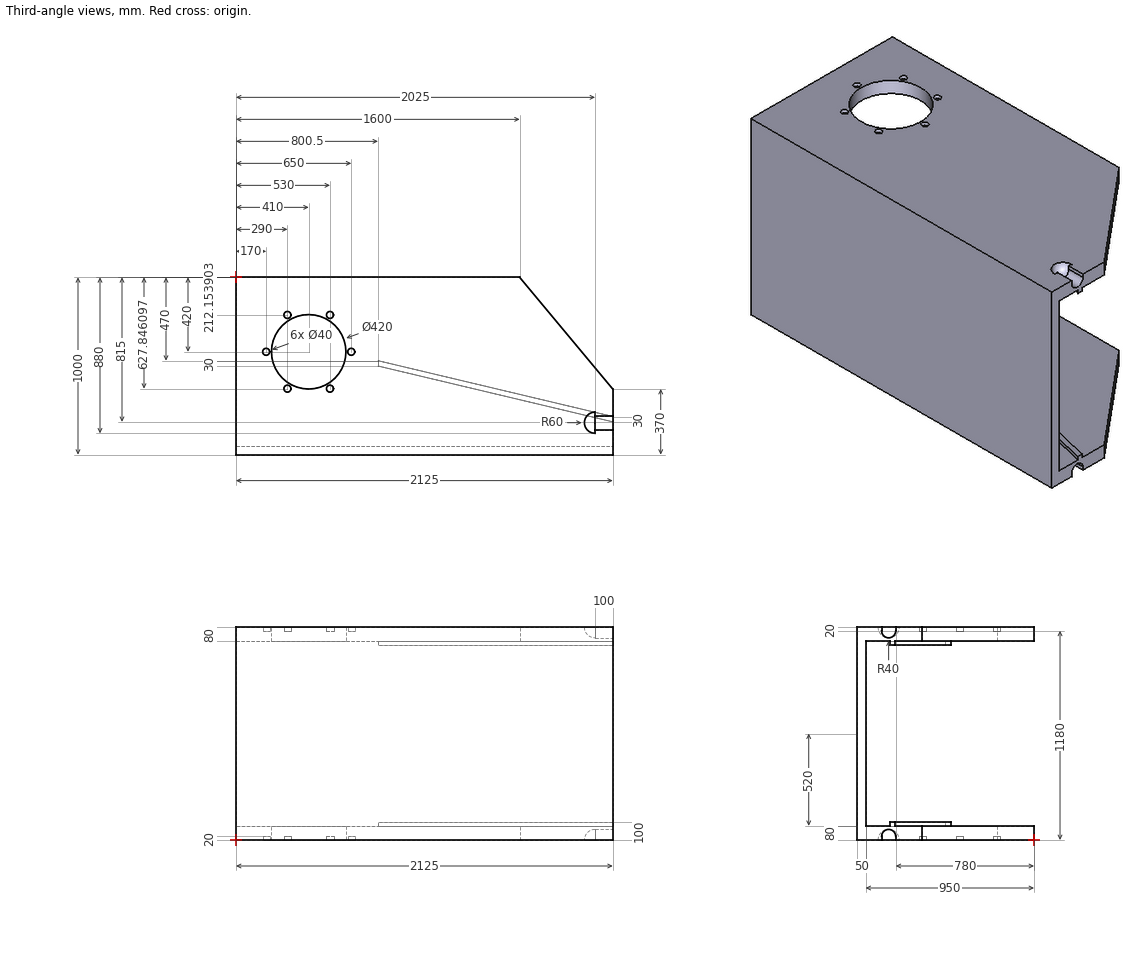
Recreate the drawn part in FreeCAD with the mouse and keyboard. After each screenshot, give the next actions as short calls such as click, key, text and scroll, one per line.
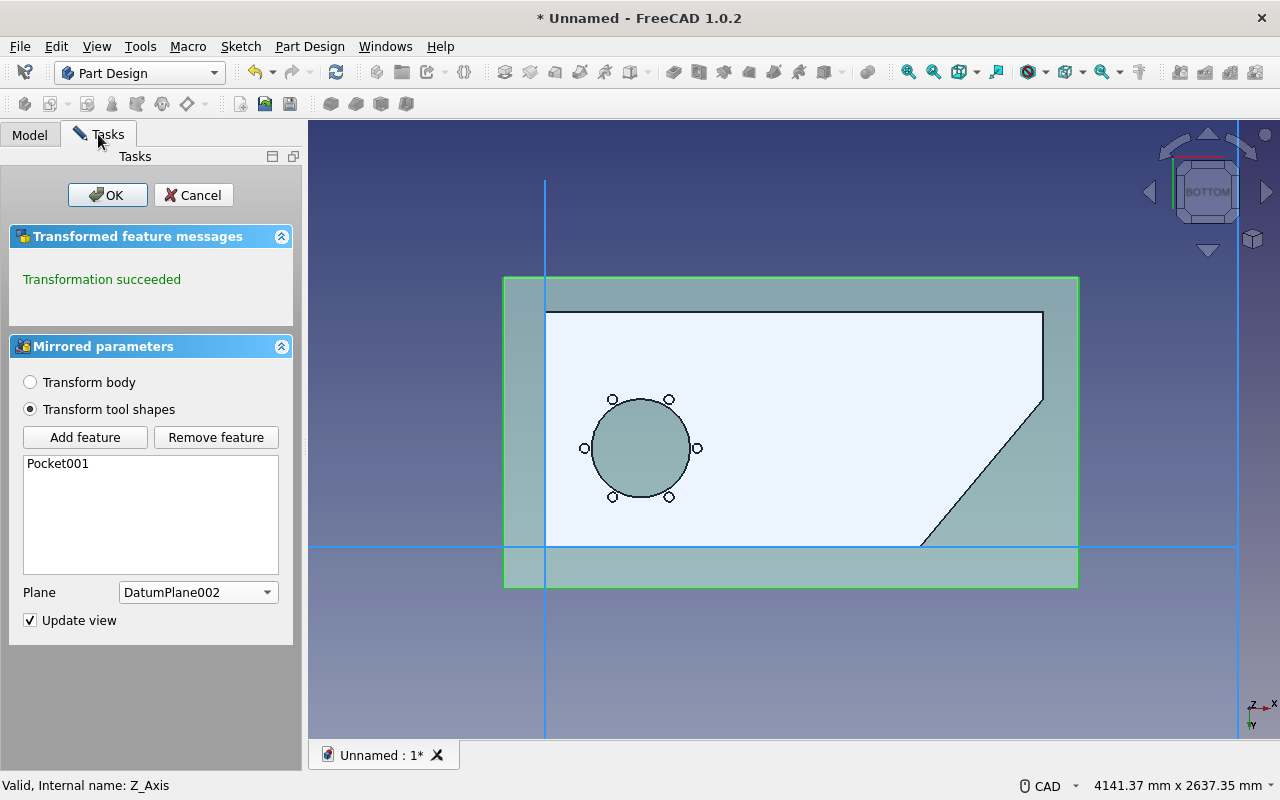
click(108, 195)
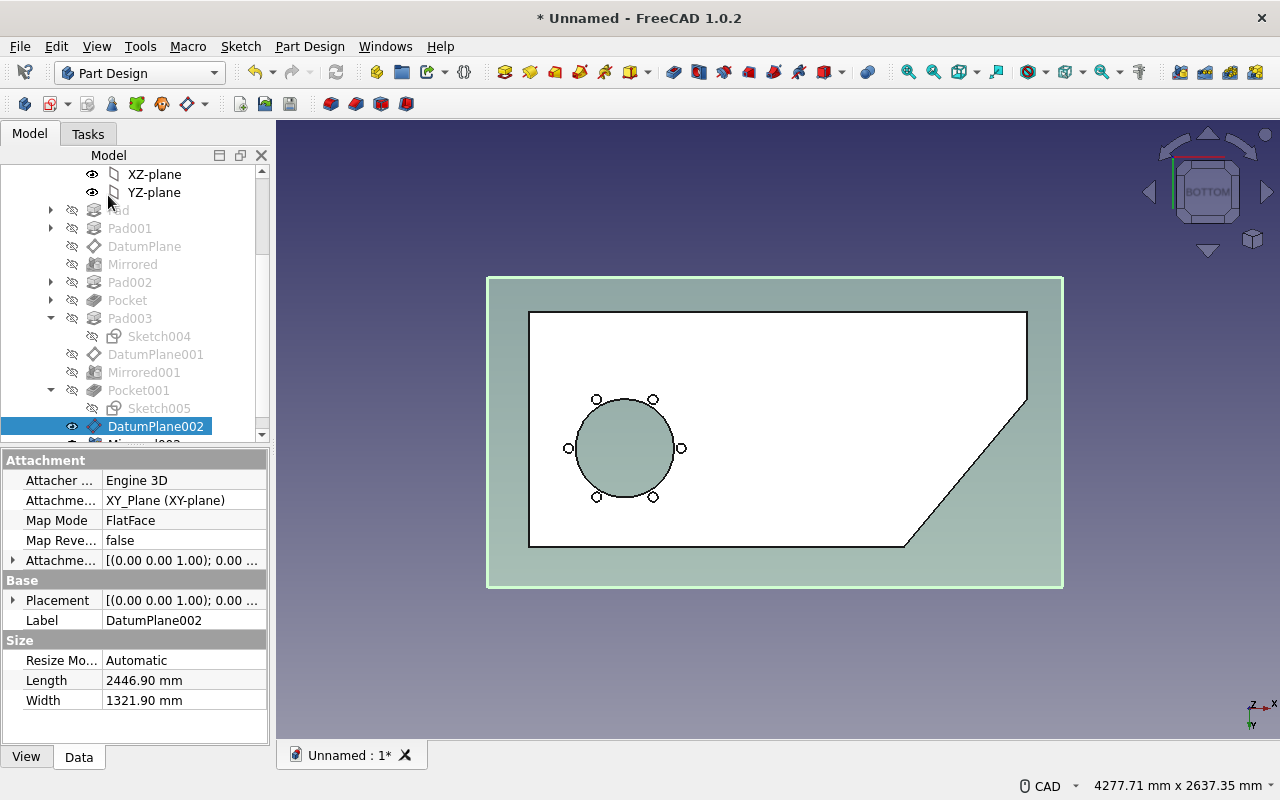
click(117, 426)
key(space)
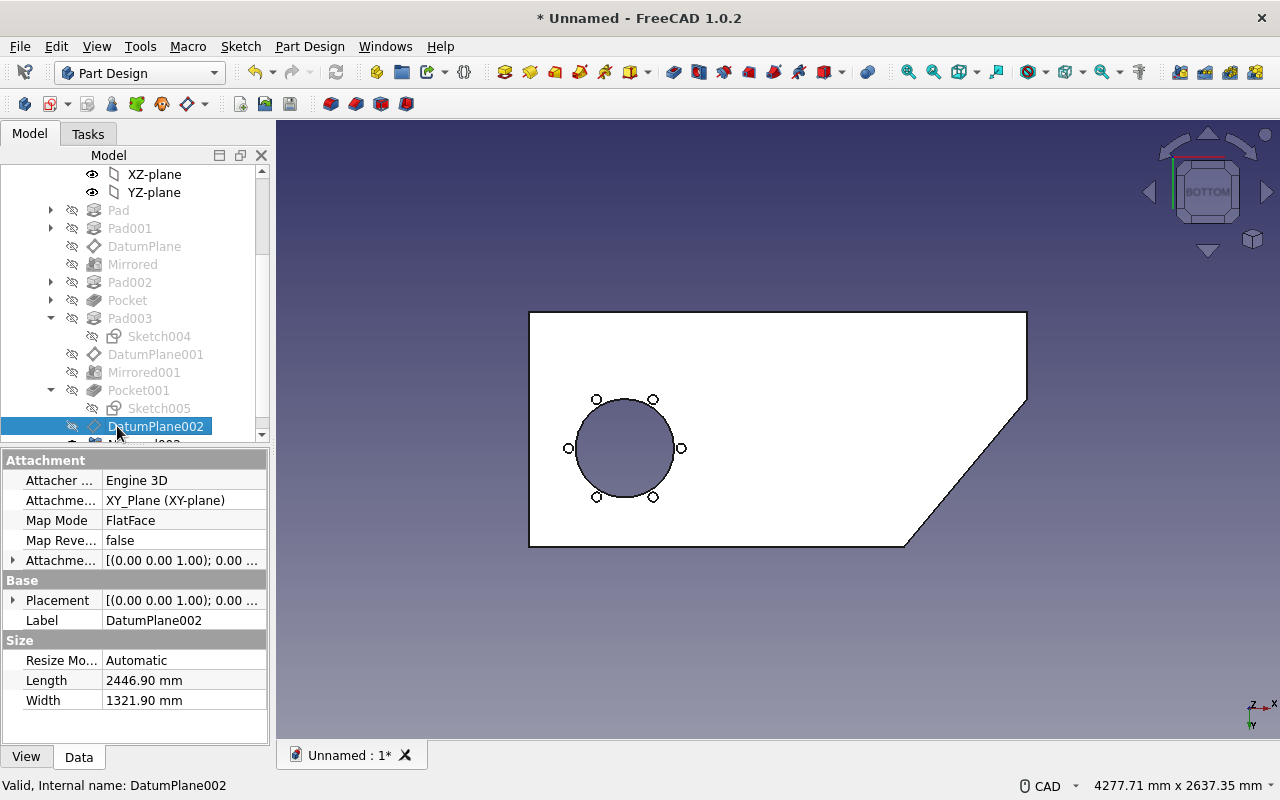
key(0)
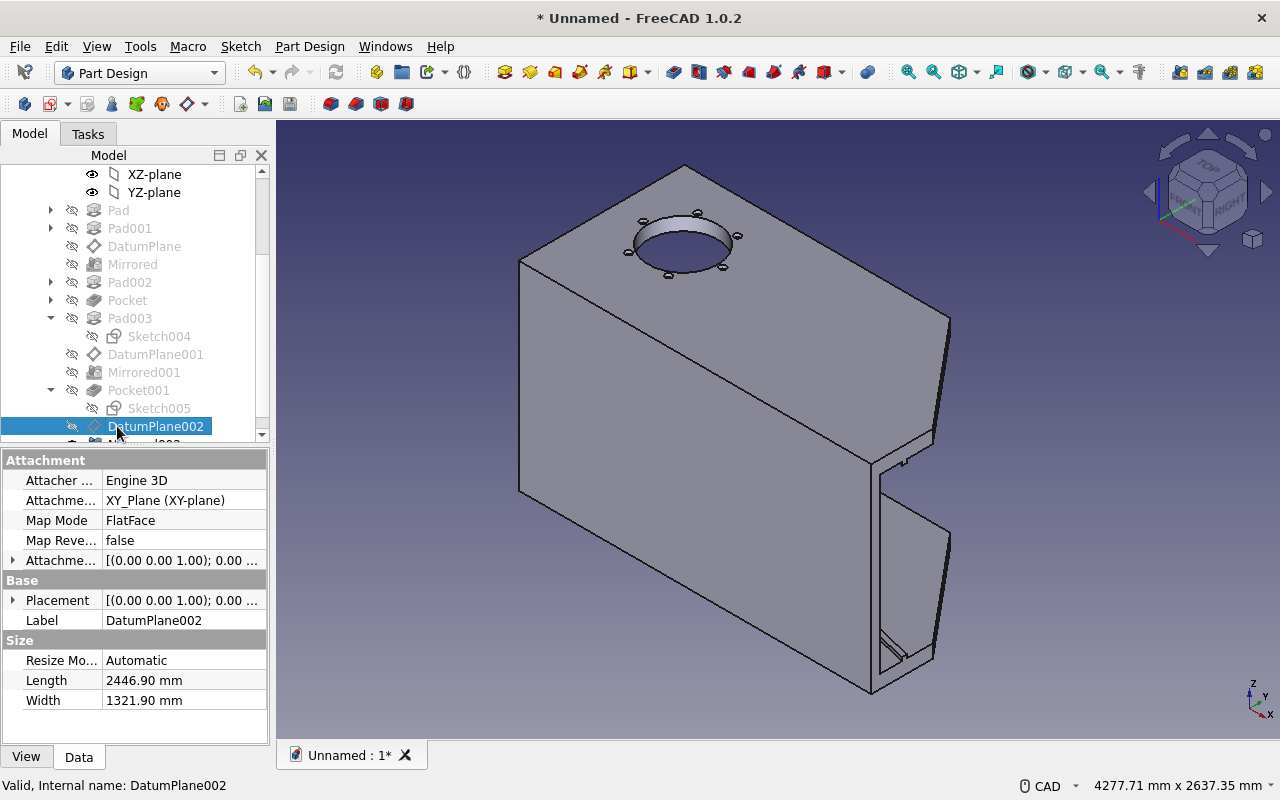
scroll(876, 477, up, 4)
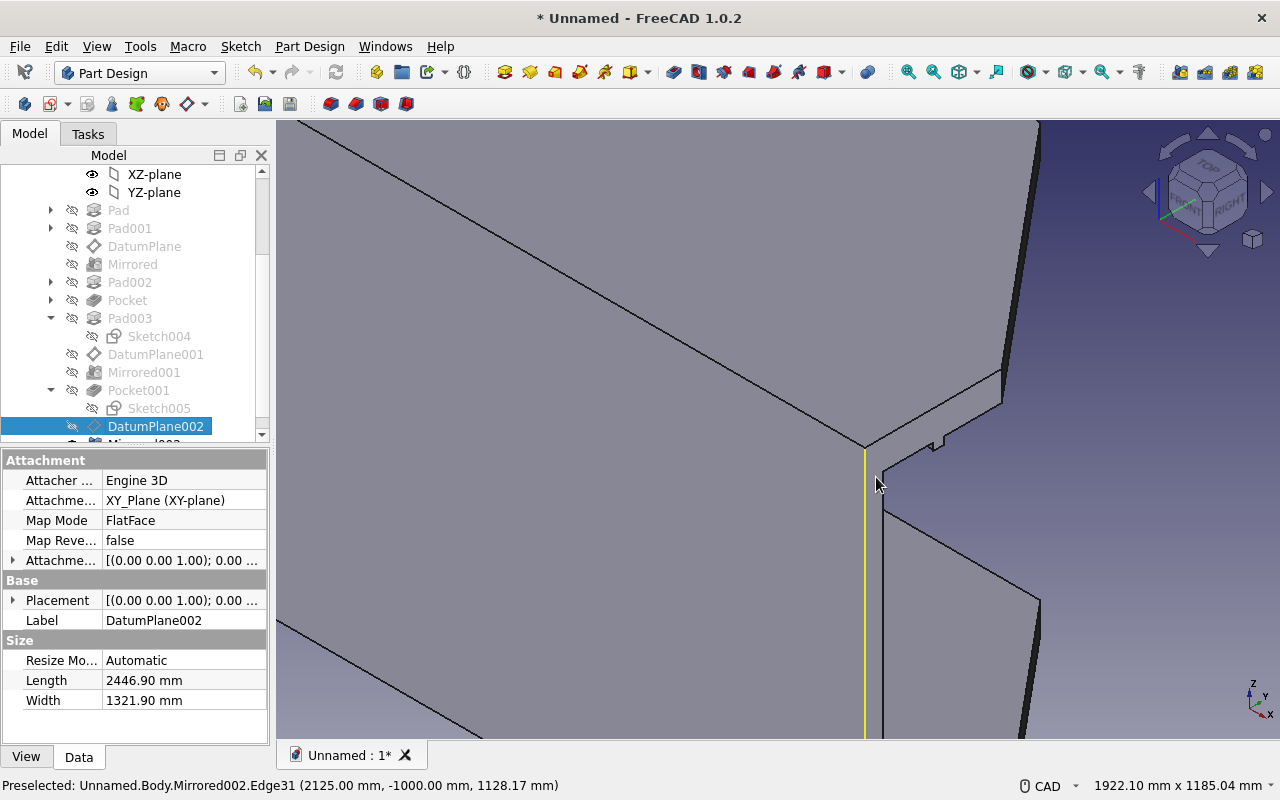
click(875, 478)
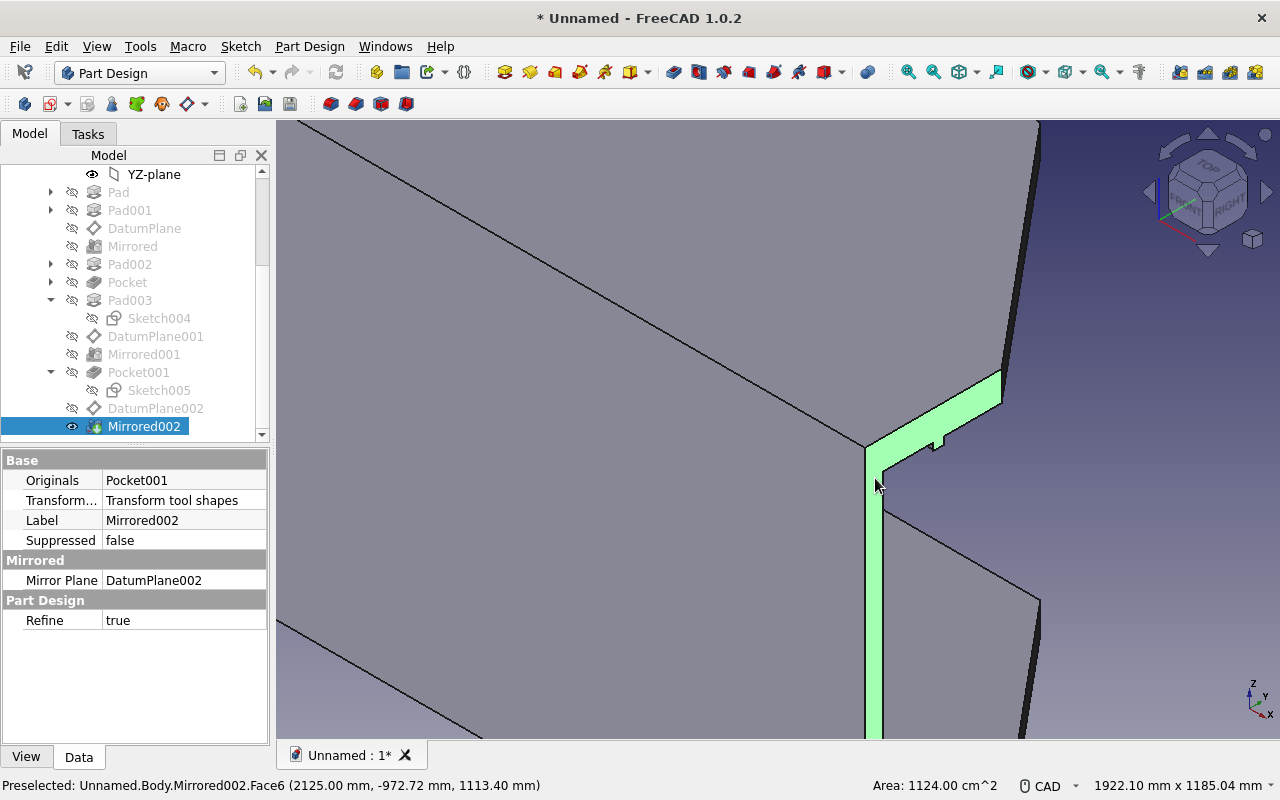
click(50, 104)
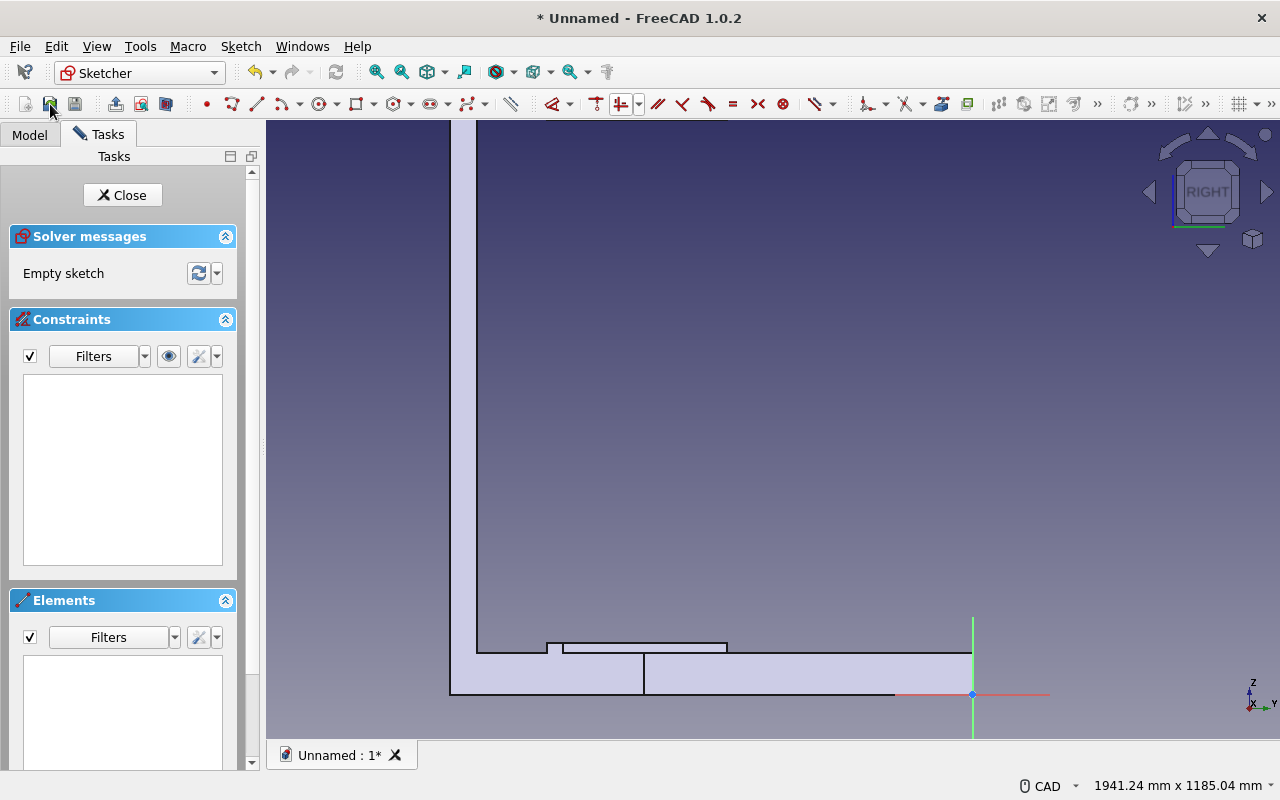
scroll(704, 430, down, 5)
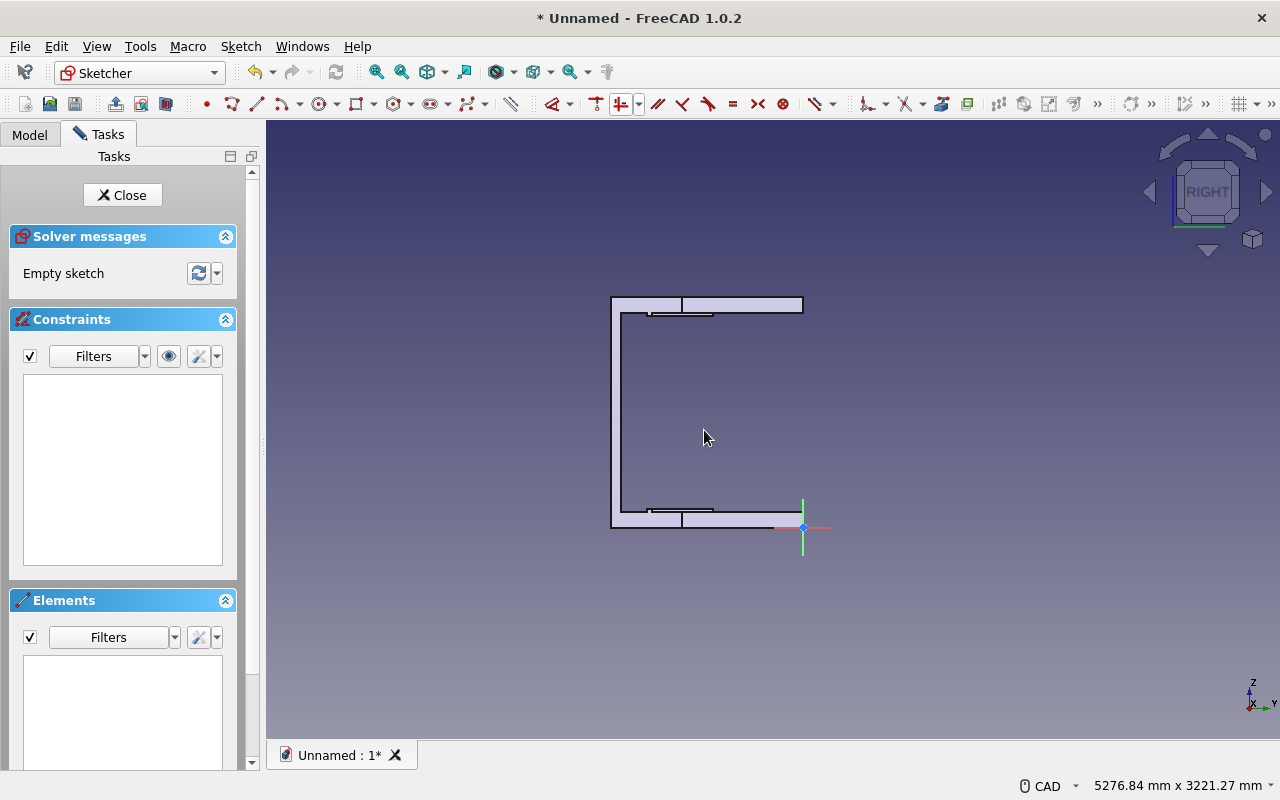
scroll(642, 296, up, 15)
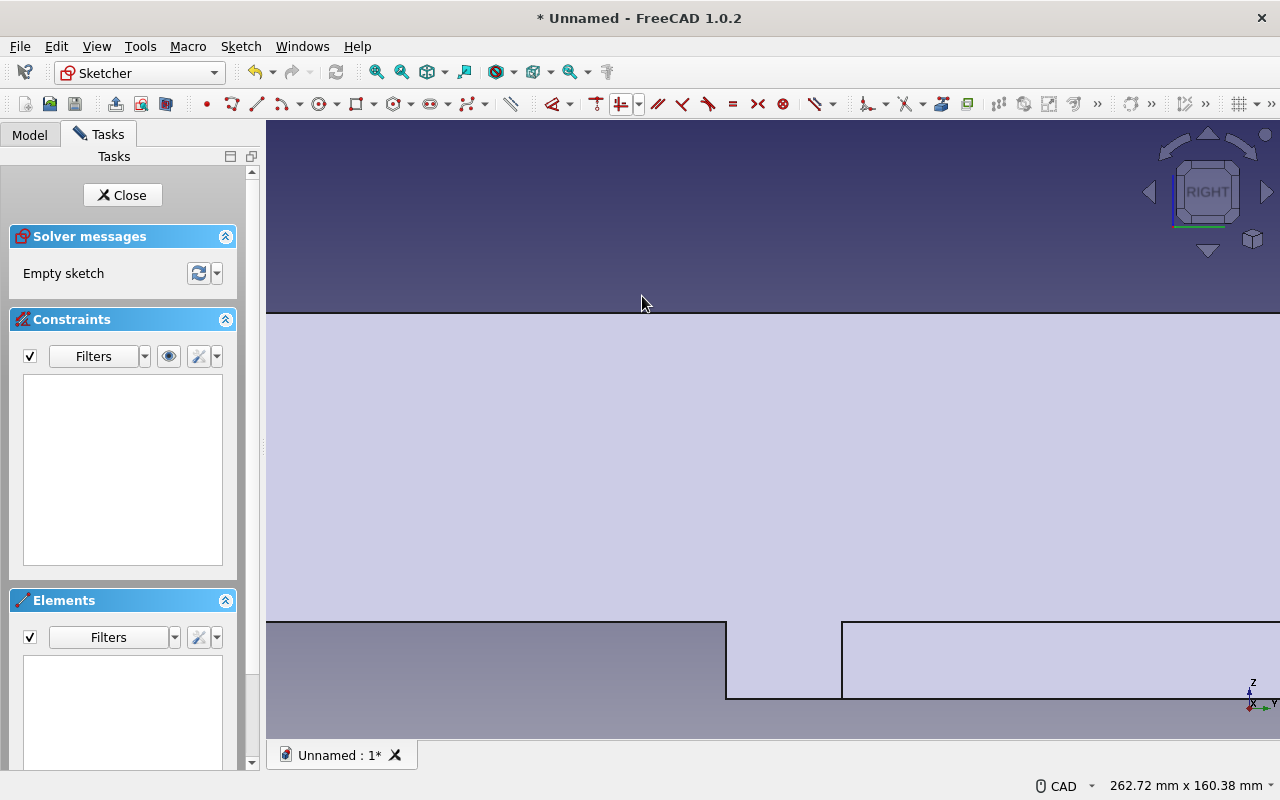
scroll(710, 429, up, 3)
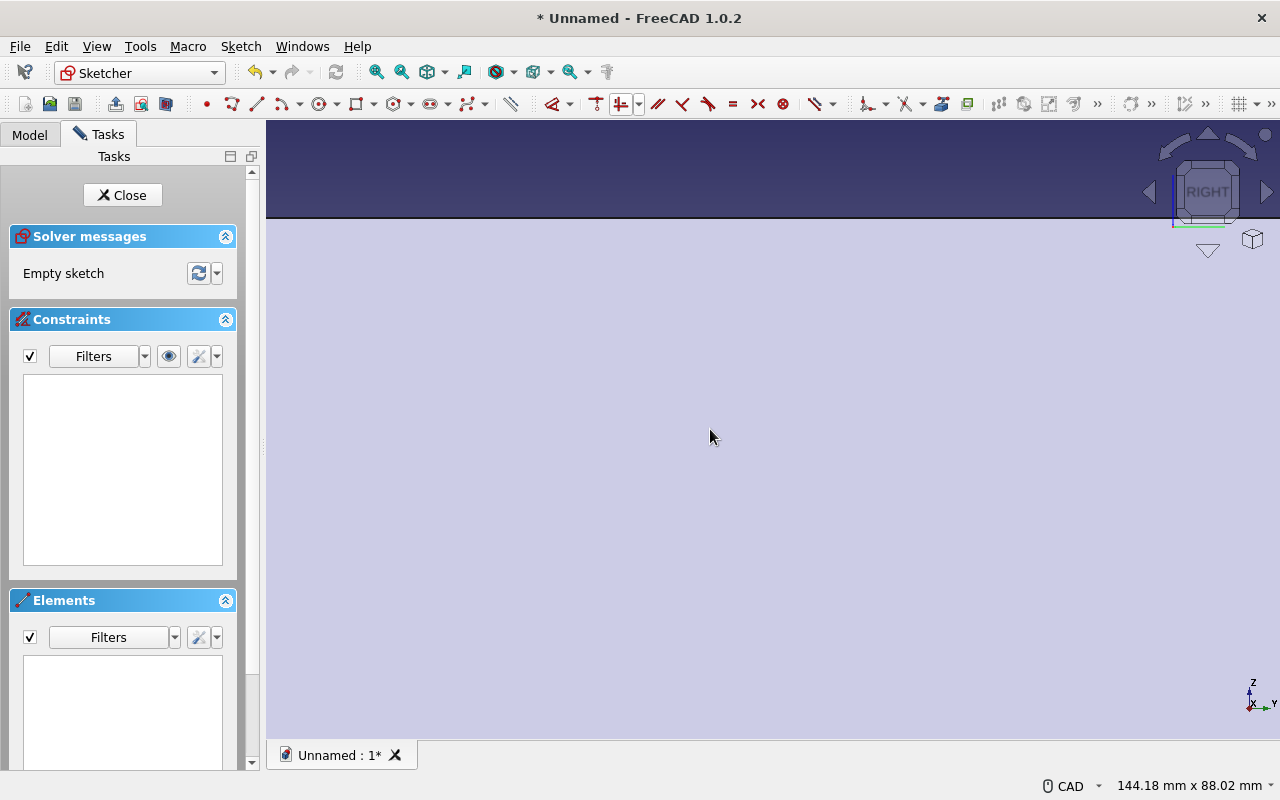
click(232, 104)